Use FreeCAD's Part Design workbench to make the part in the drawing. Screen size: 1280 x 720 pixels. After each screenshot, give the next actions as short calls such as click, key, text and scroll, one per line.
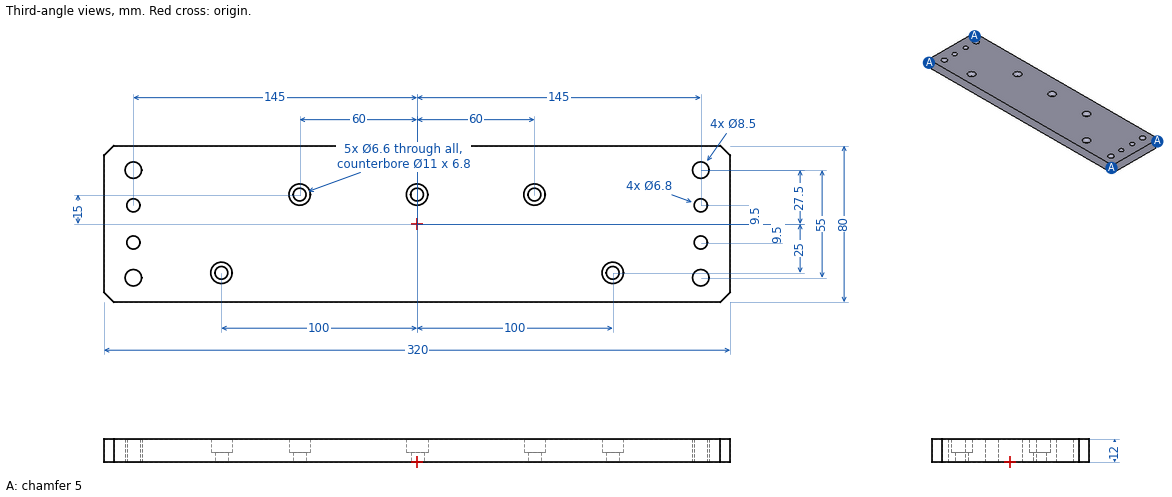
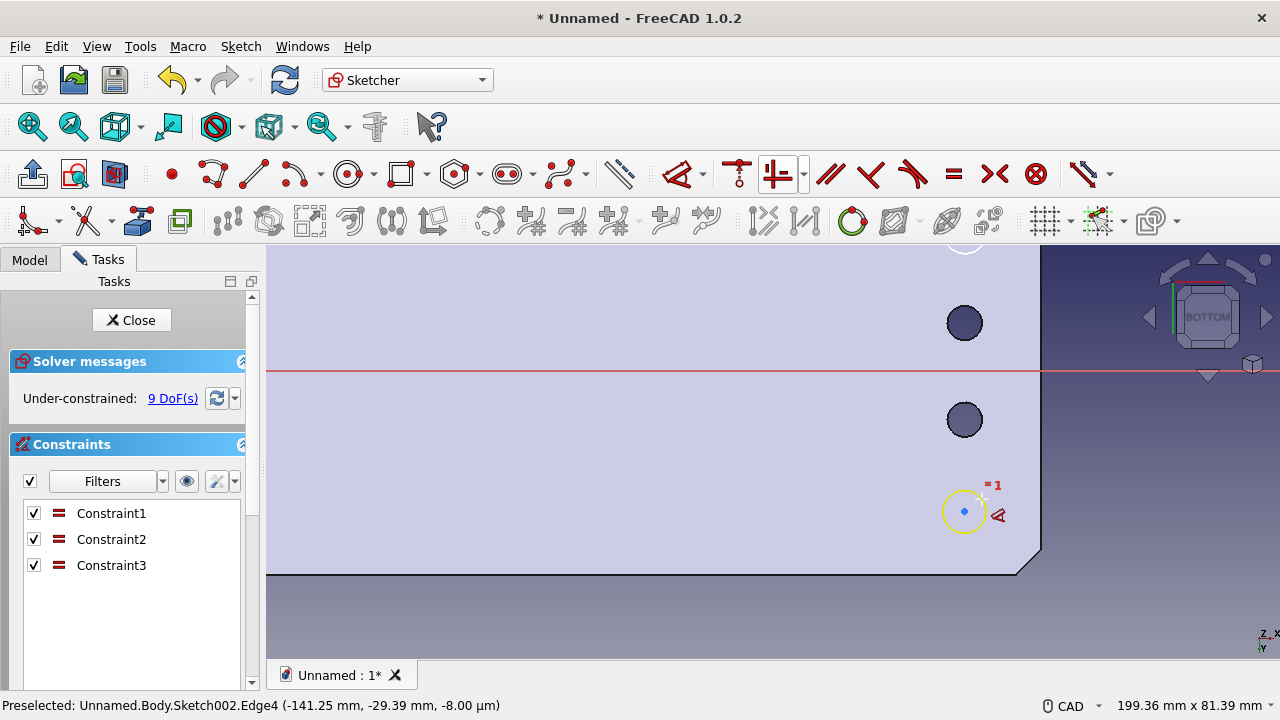
click(980, 497)
click(1003, 475)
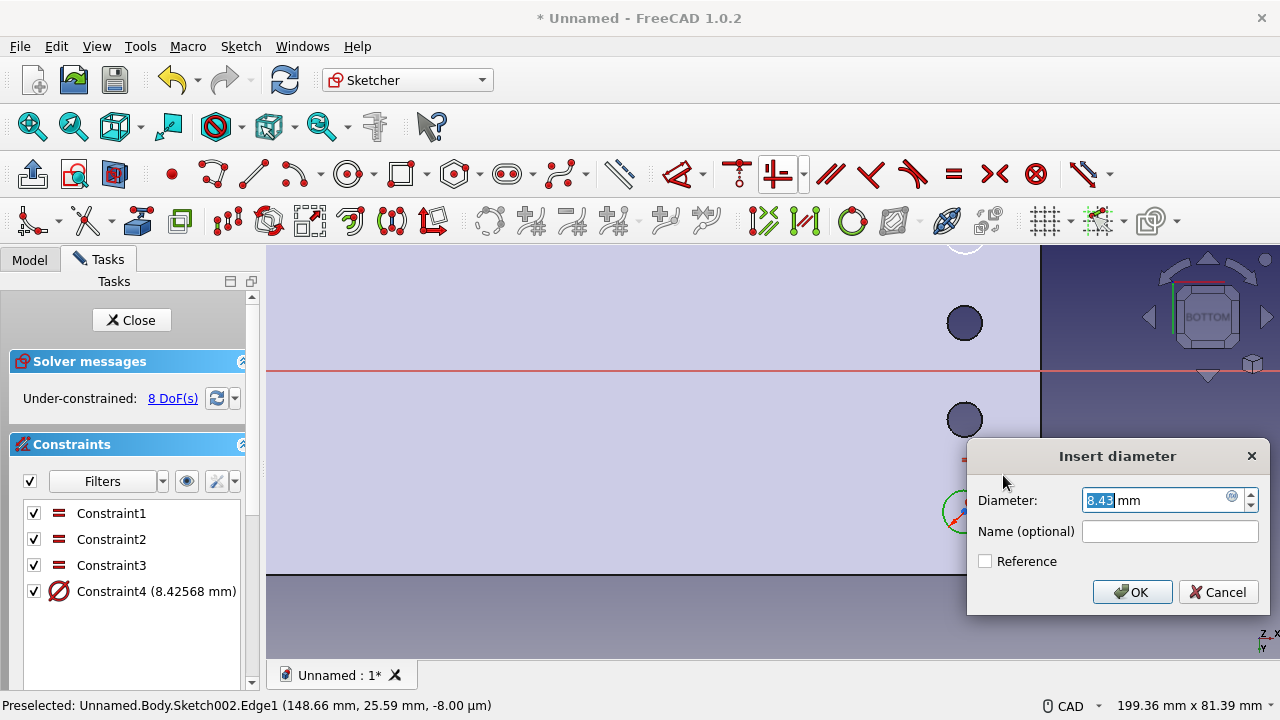
text(8.5)
key(Return)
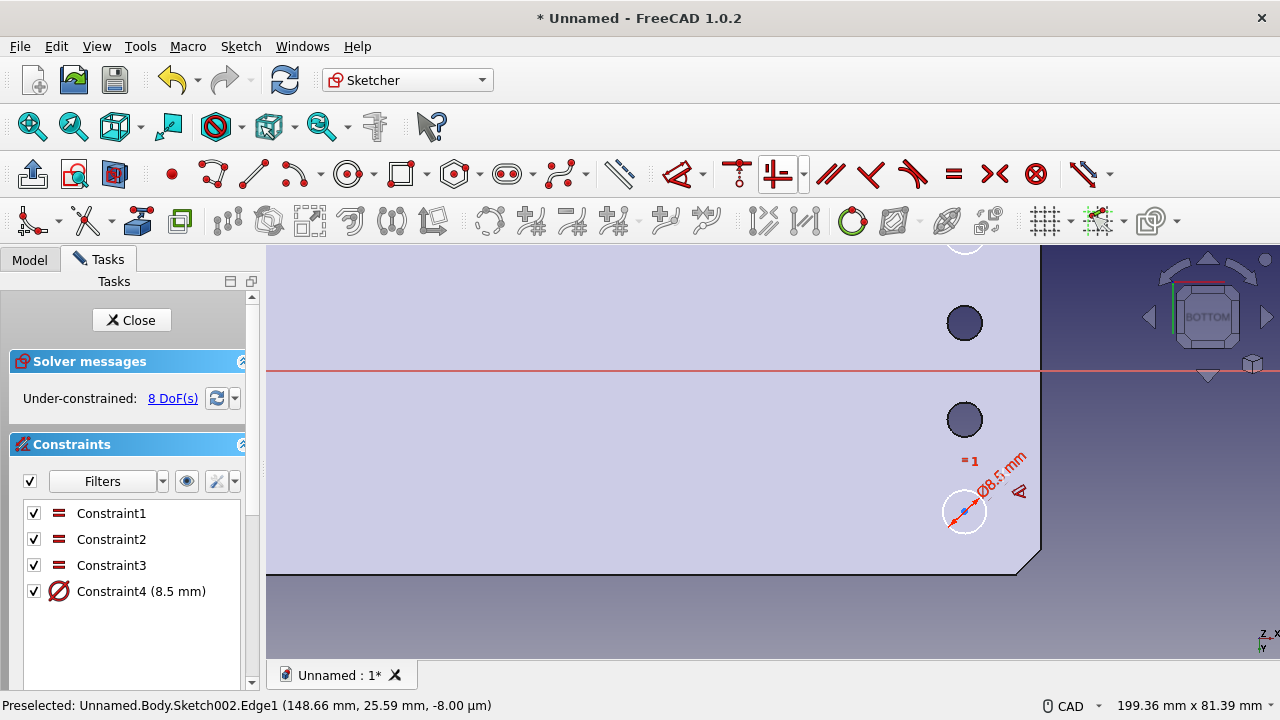
click(965, 512)
click(629, 546)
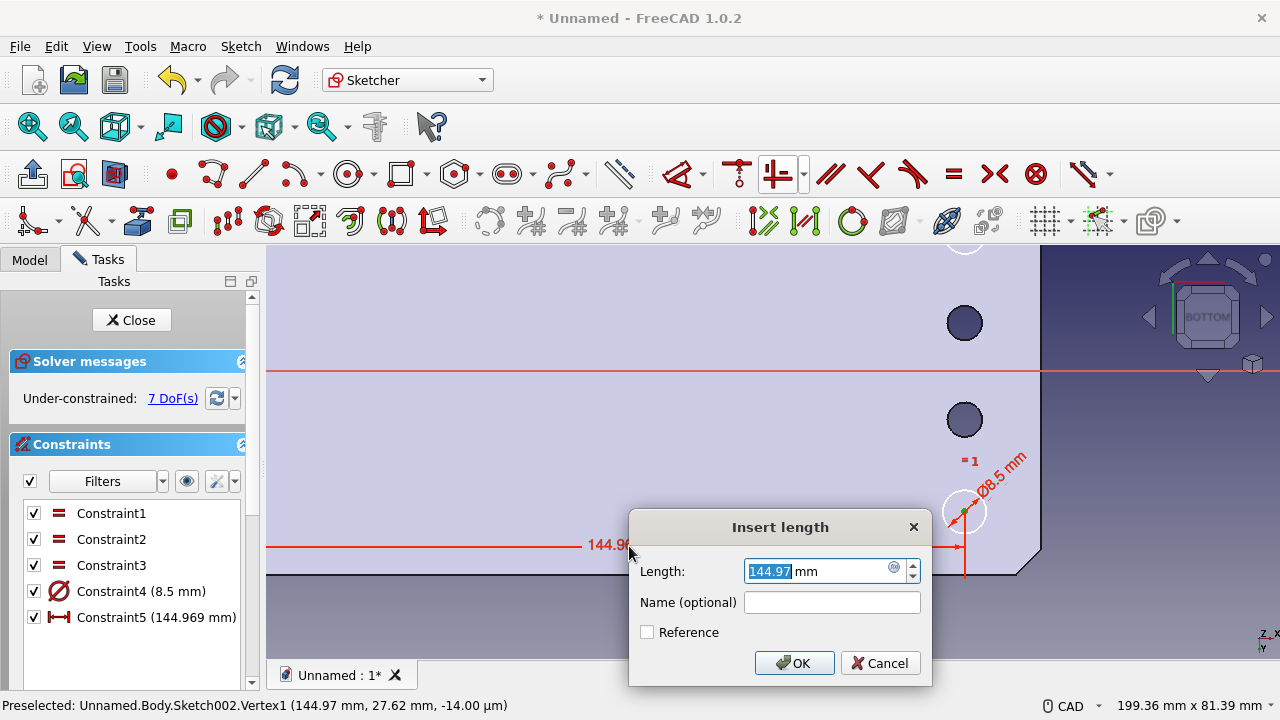
text(145)
key(Return)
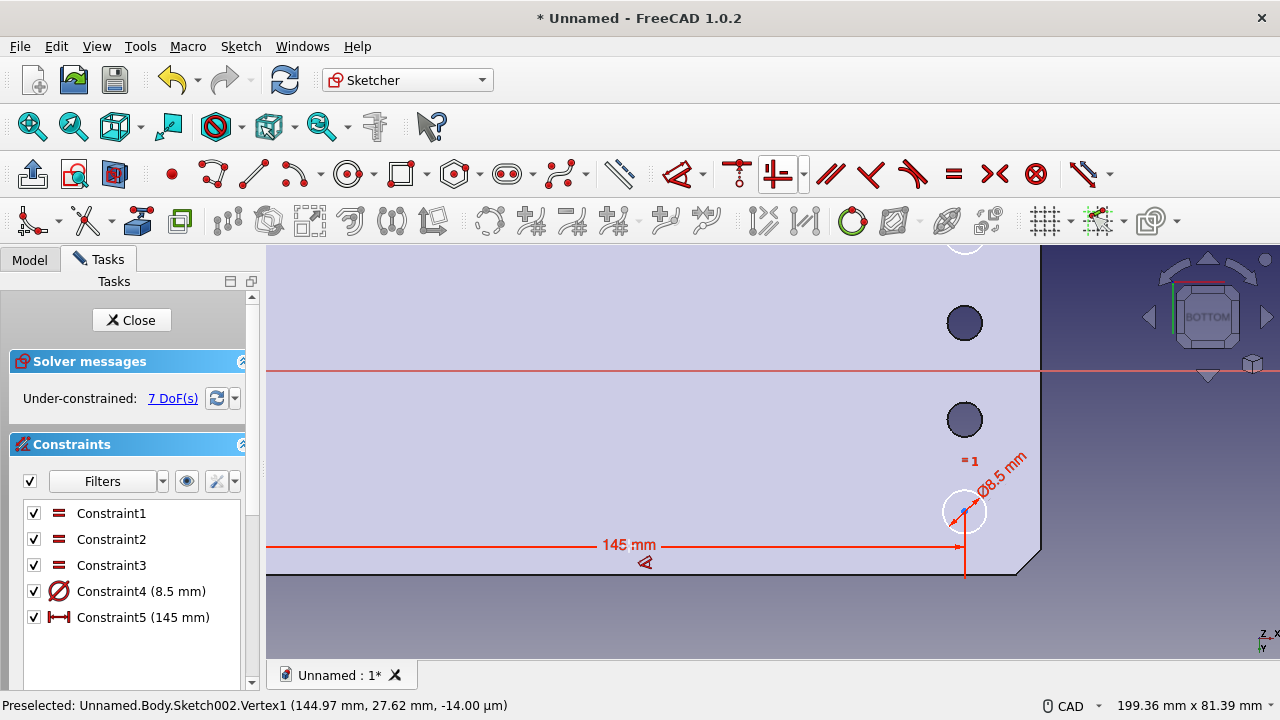
scroll(982, 499, down, 5)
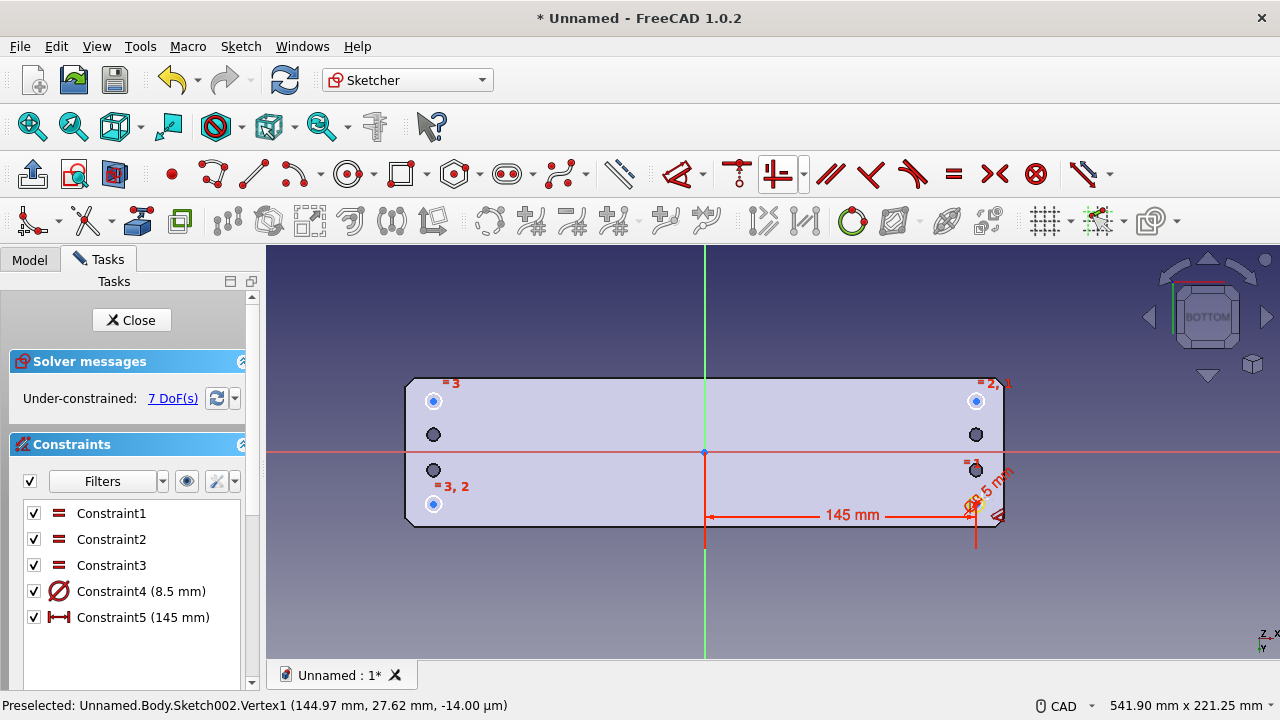
click(976, 401)
click(841, 367)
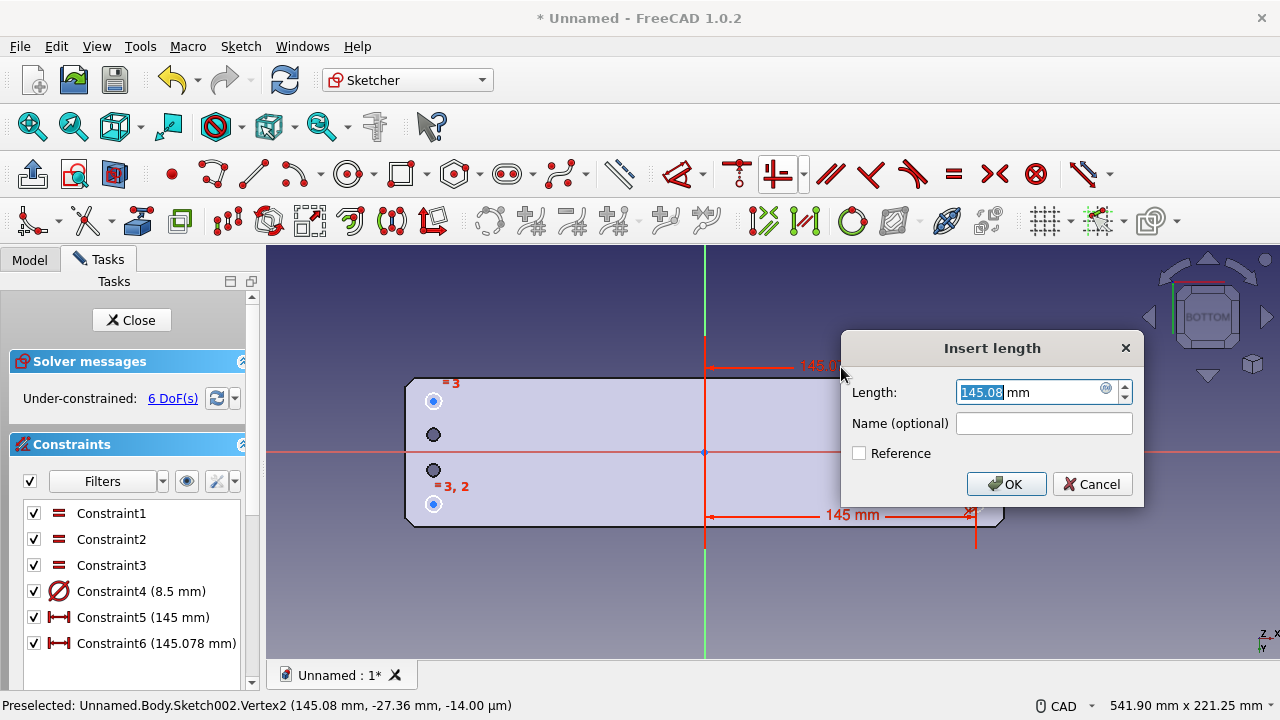
text(145)
key(Return)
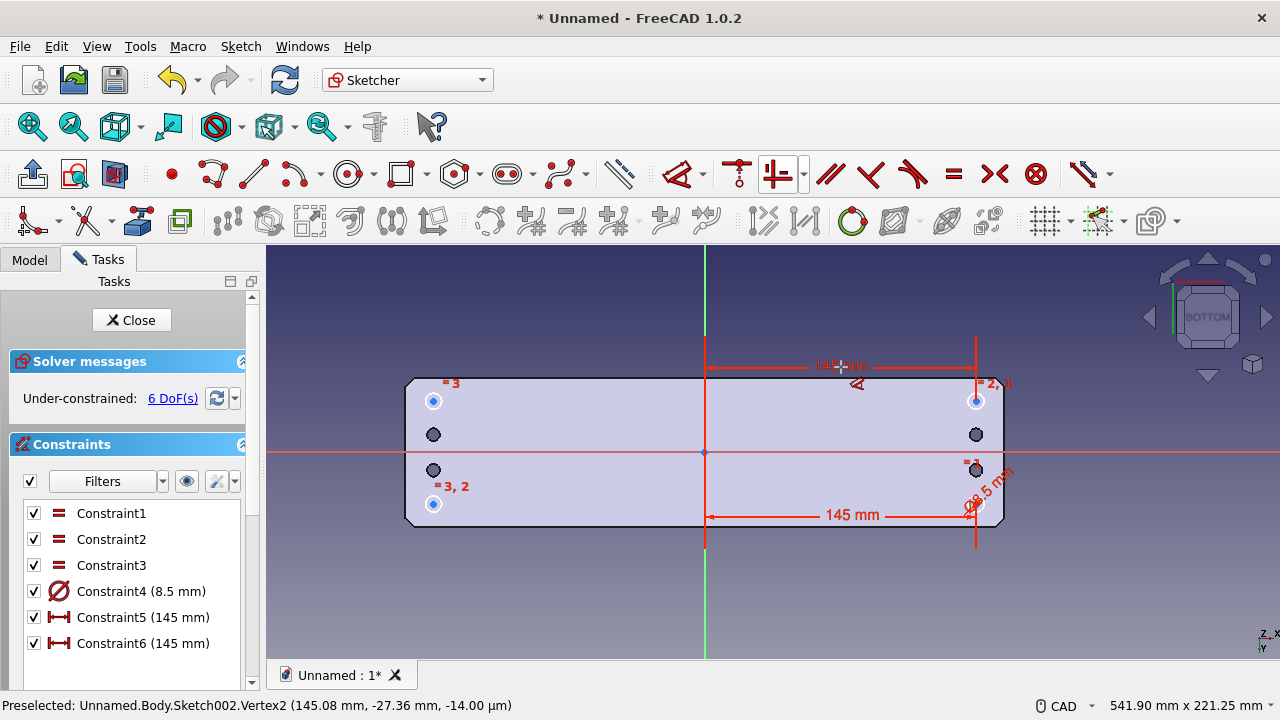
click(434, 504)
click(569, 538)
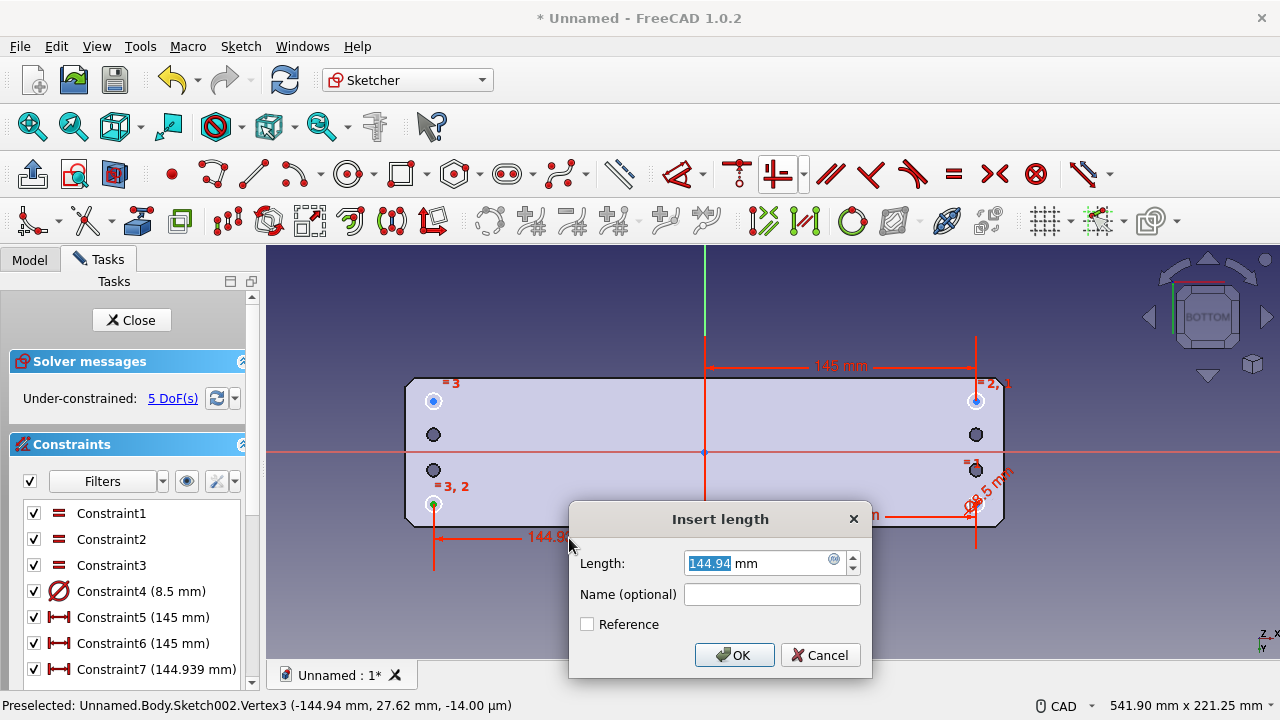
text(145)
key(Return)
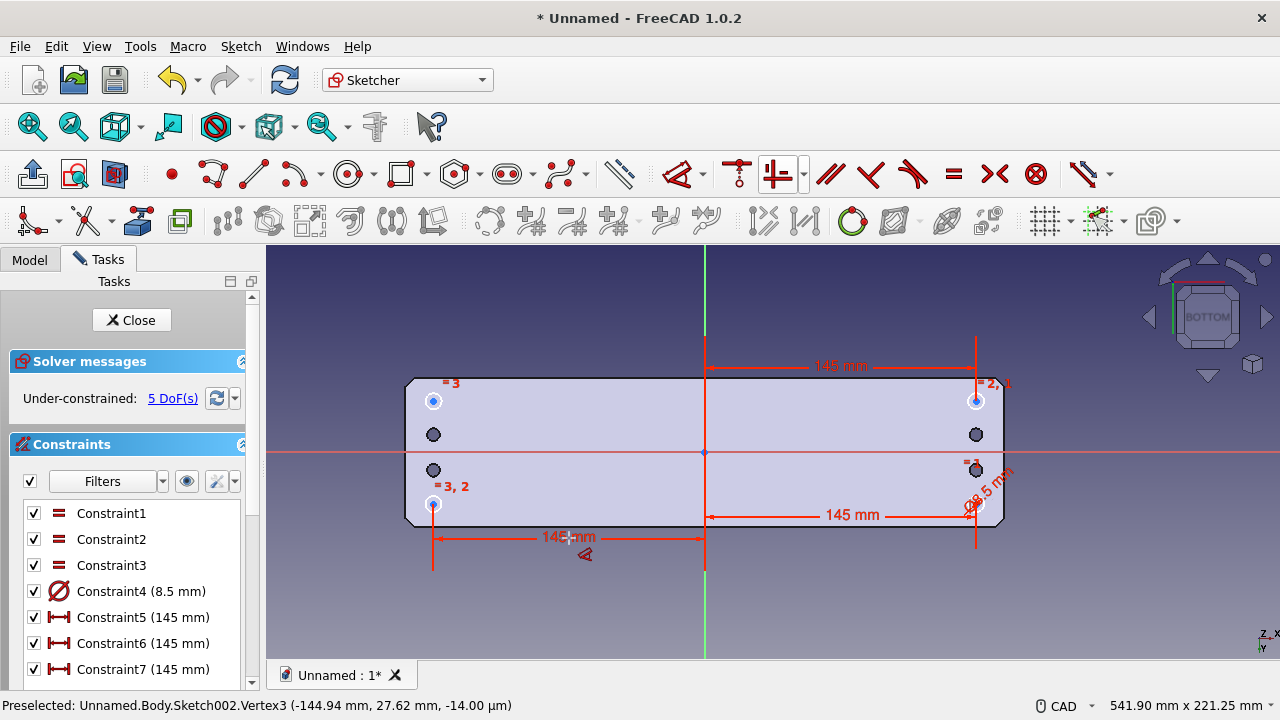
click(434, 401)
click(569, 367)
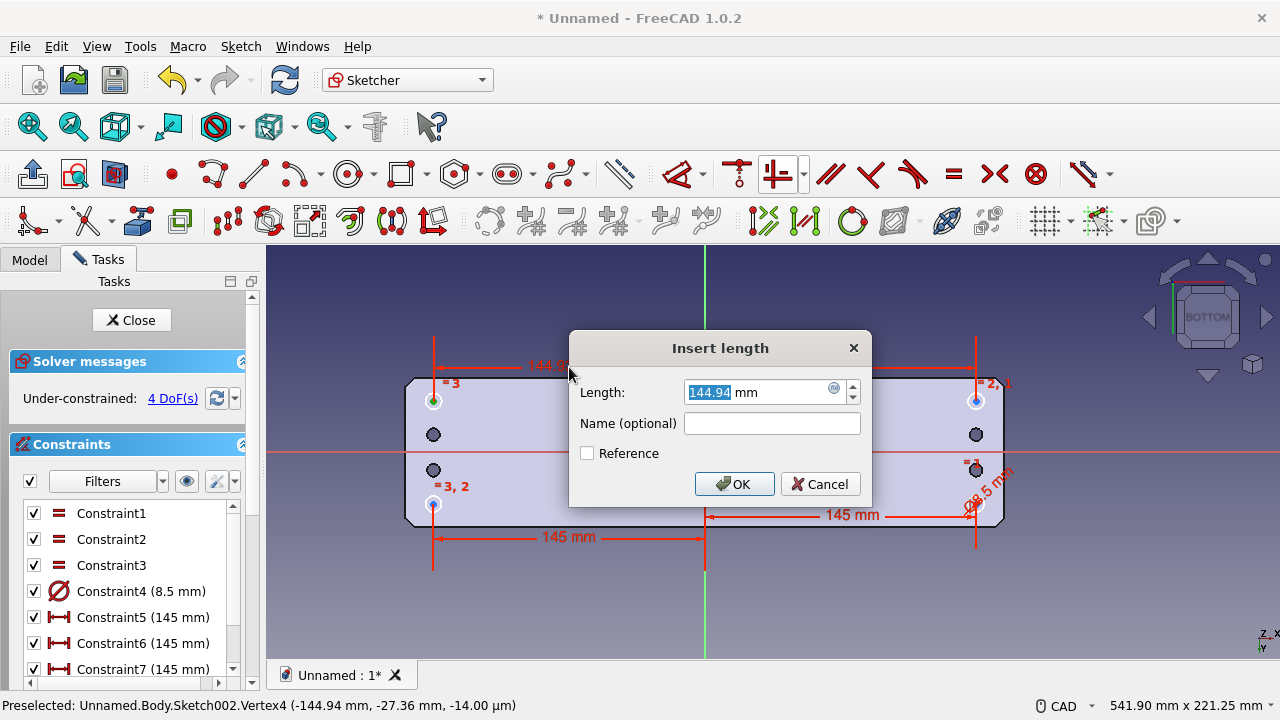
text(145)
key(Return)